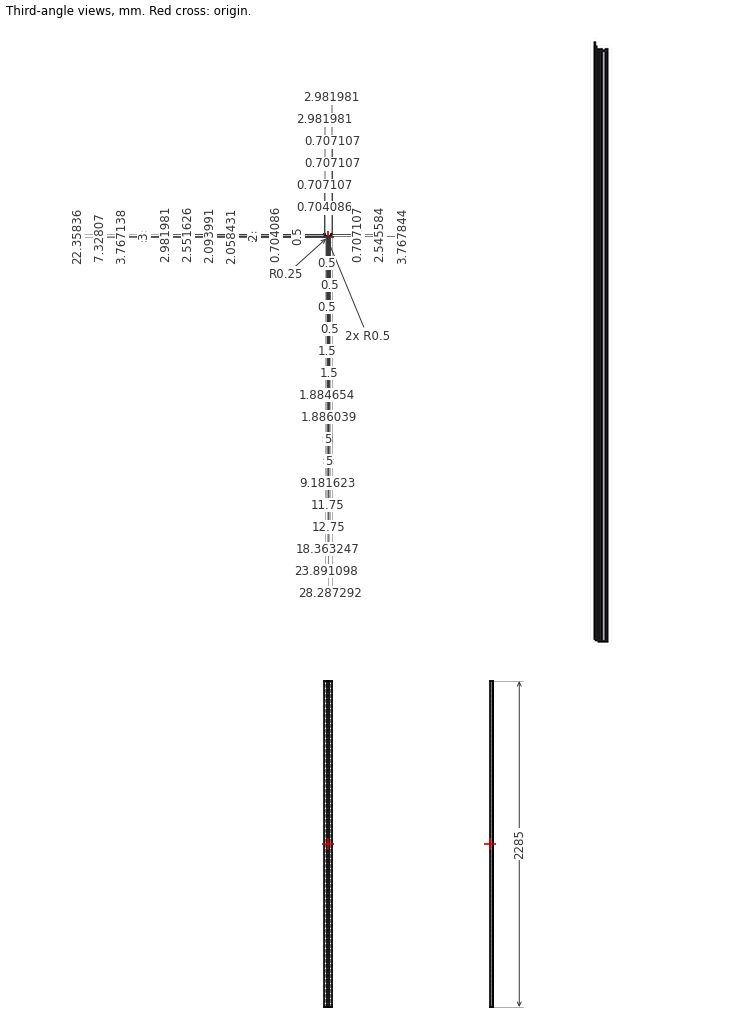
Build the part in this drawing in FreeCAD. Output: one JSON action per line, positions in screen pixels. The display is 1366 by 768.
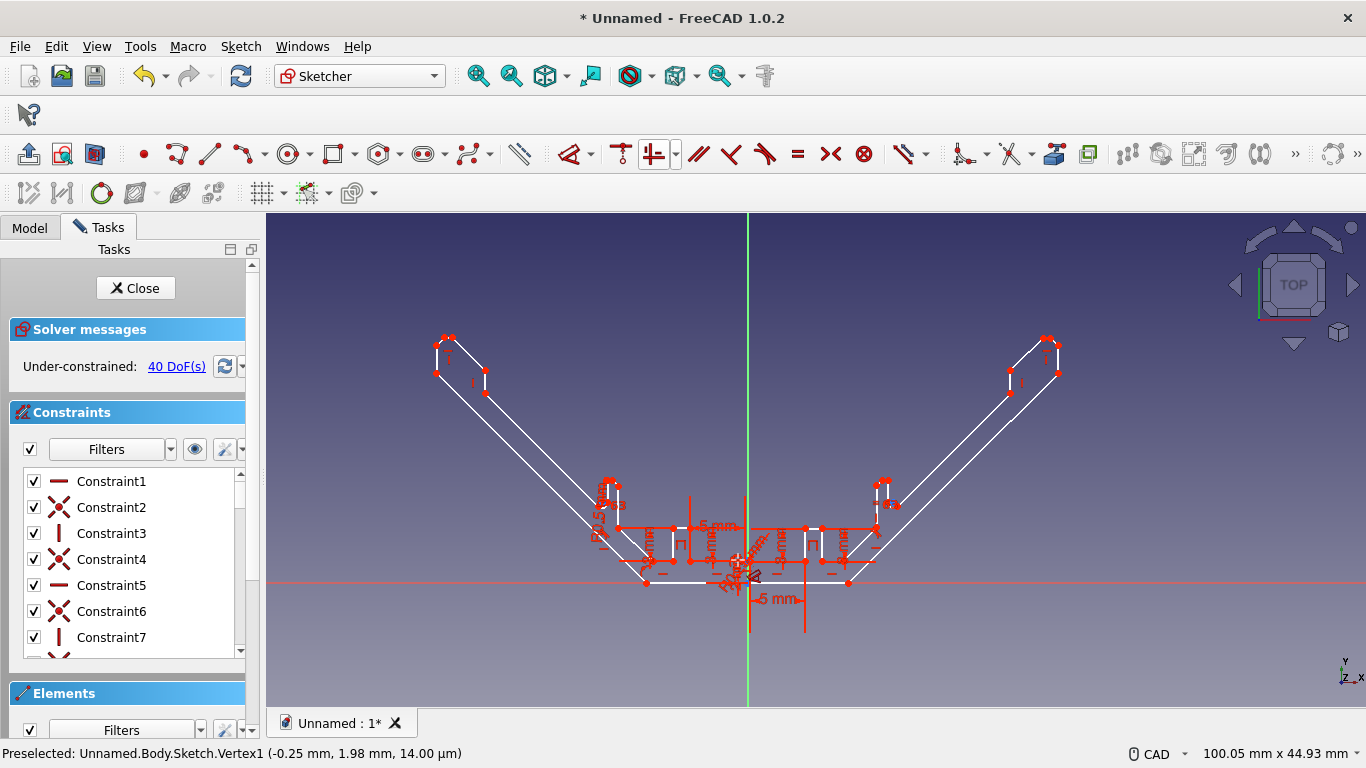
{"action": "scroll", "coordinate": [843, 562], "scroll_direction": "up", "scroll_amount": 3}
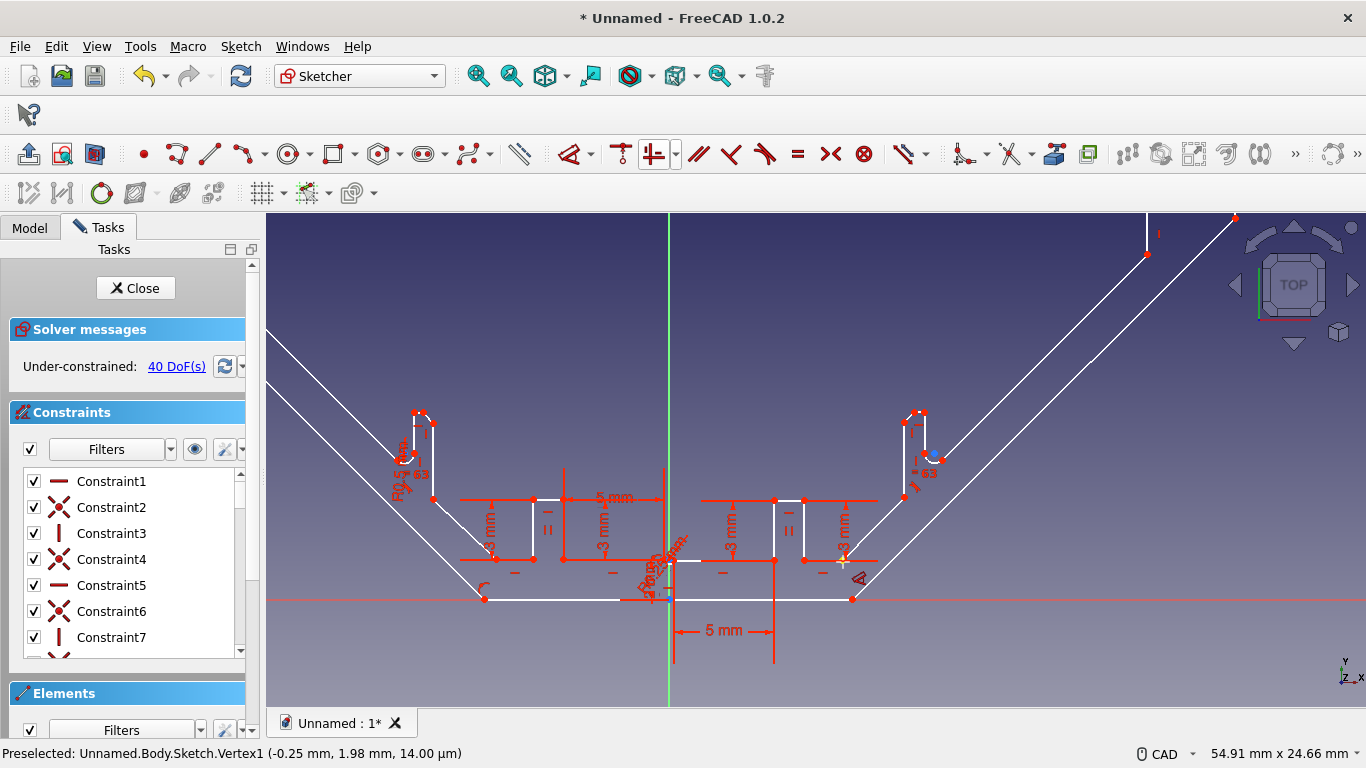
{"action": "left_click", "coordinate": [843, 561]}
{"action": "left_click", "coordinate": [901, 580]}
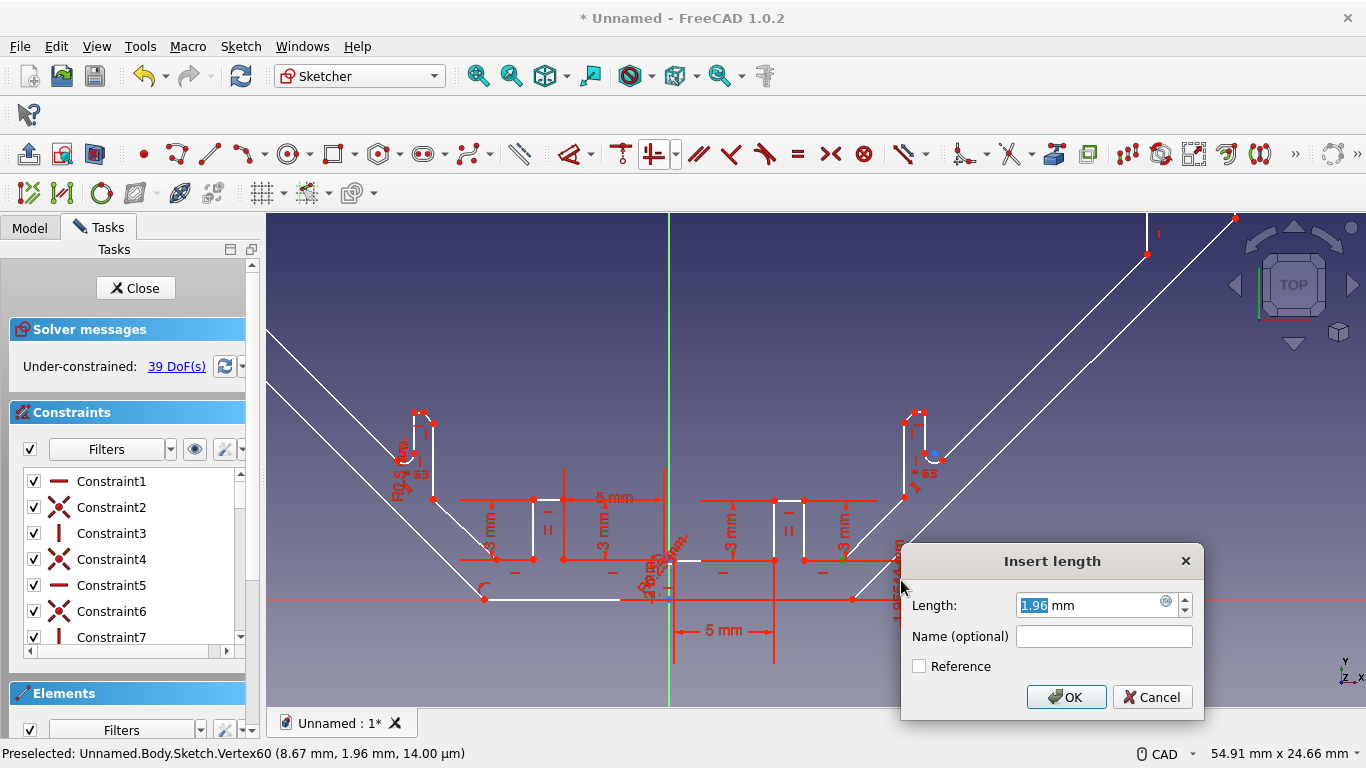
{"action": "type", "text": "2"}
{"action": "key", "text": "Return"}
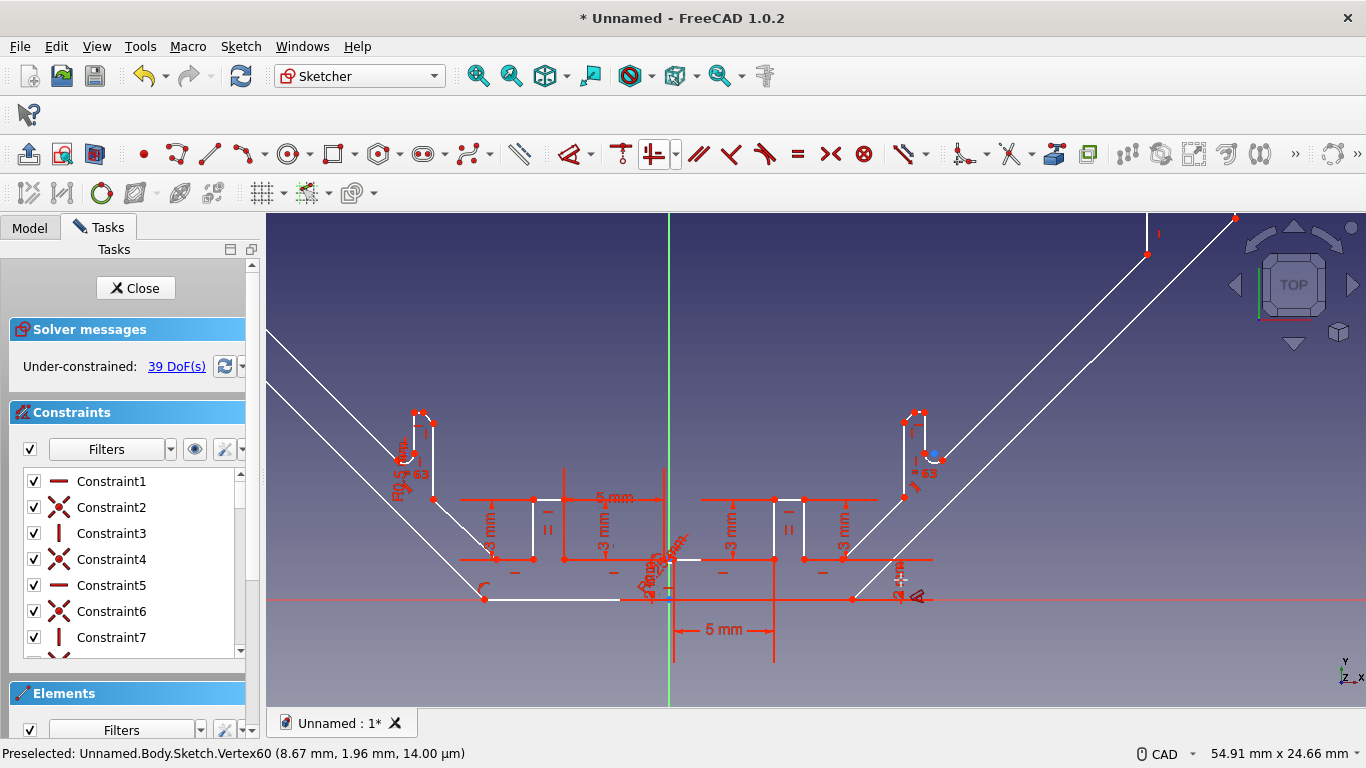
{"action": "scroll", "coordinate": [669, 558], "scroll_direction": "up", "scroll_amount": 5}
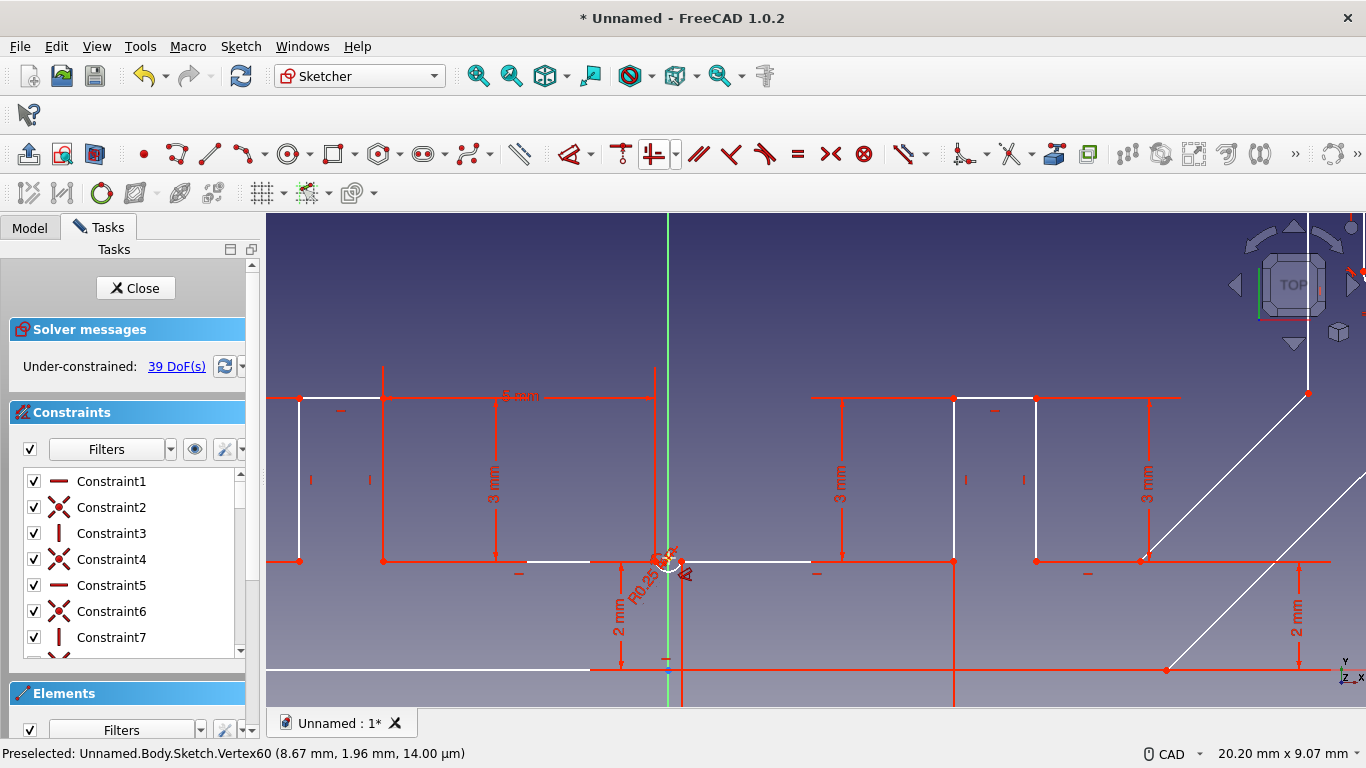
{"action": "left_click", "coordinate": [668, 558]}
{"action": "left_click", "coordinate": [634, 640]}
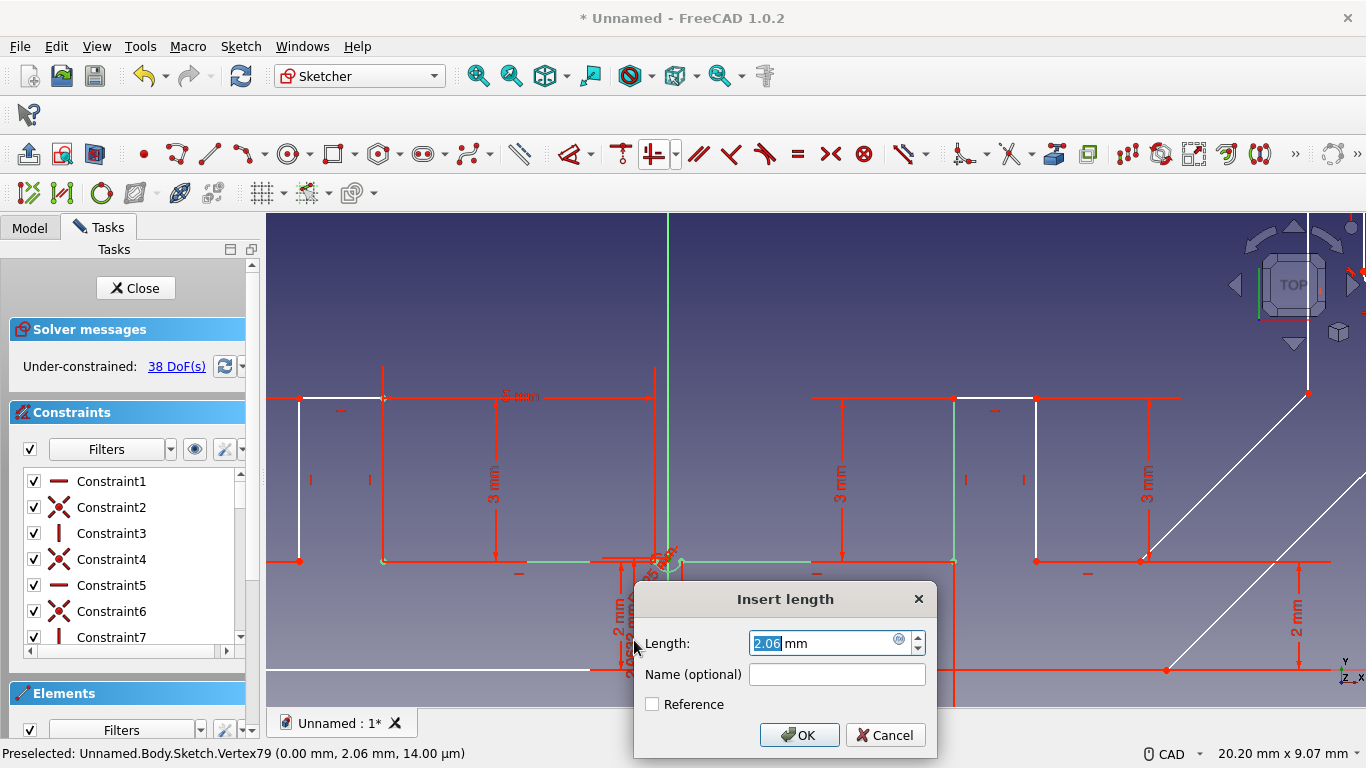
{"action": "type", "text": "2"}
{"action": "key", "text": "Return"}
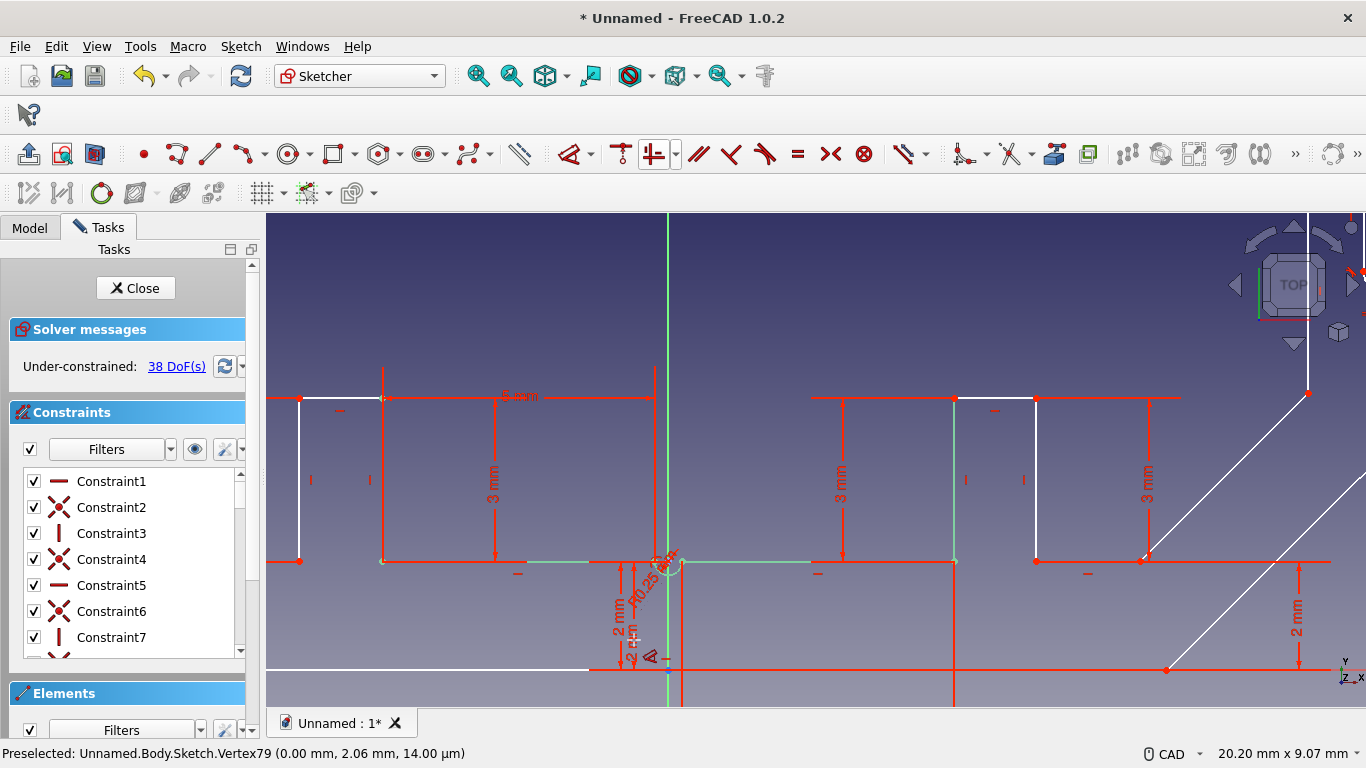
{"action": "left_click", "coordinate": [358, 398]}
{"action": "left_click", "coordinate": [341, 432]}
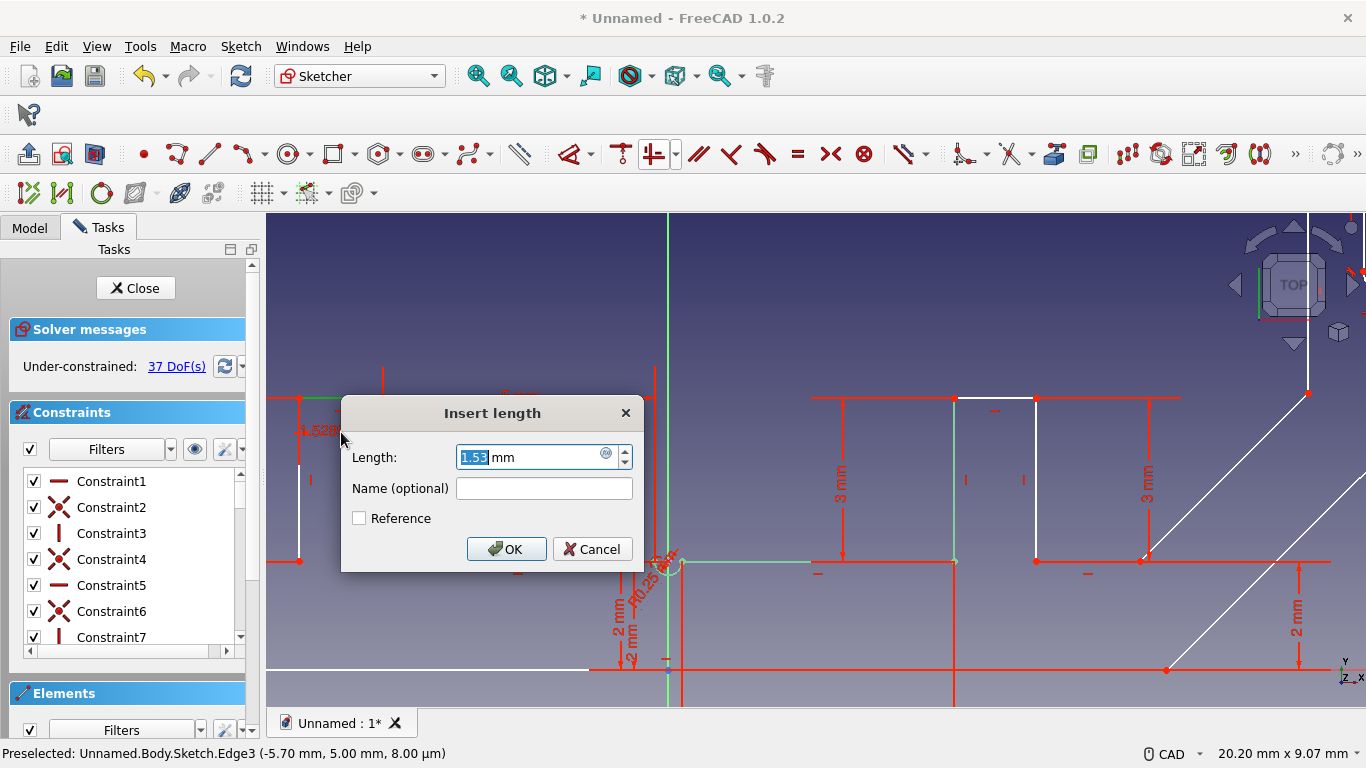
{"action": "type", "text": "1.5"}
{"action": "key", "text": "Return"}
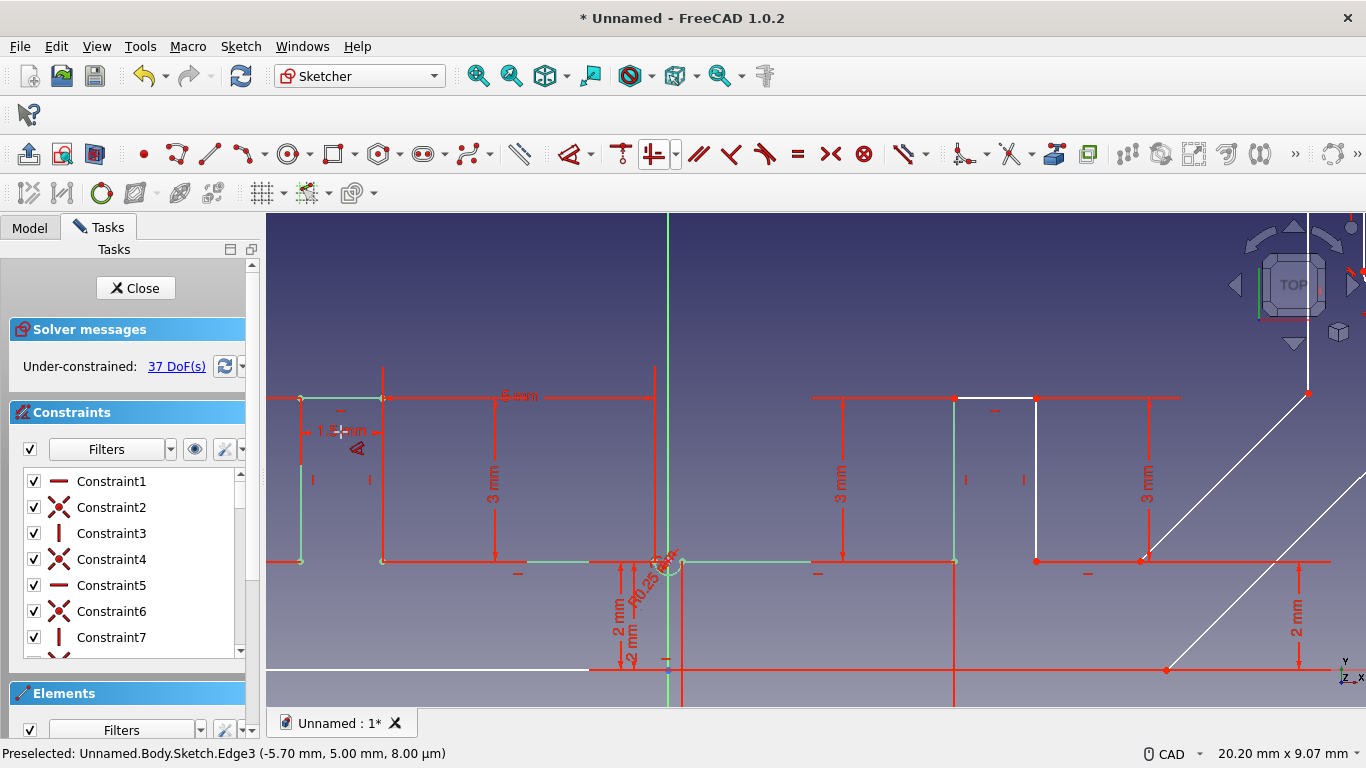
{"action": "scroll", "coordinate": [767, 561], "scroll_direction": "down", "scroll_amount": 8}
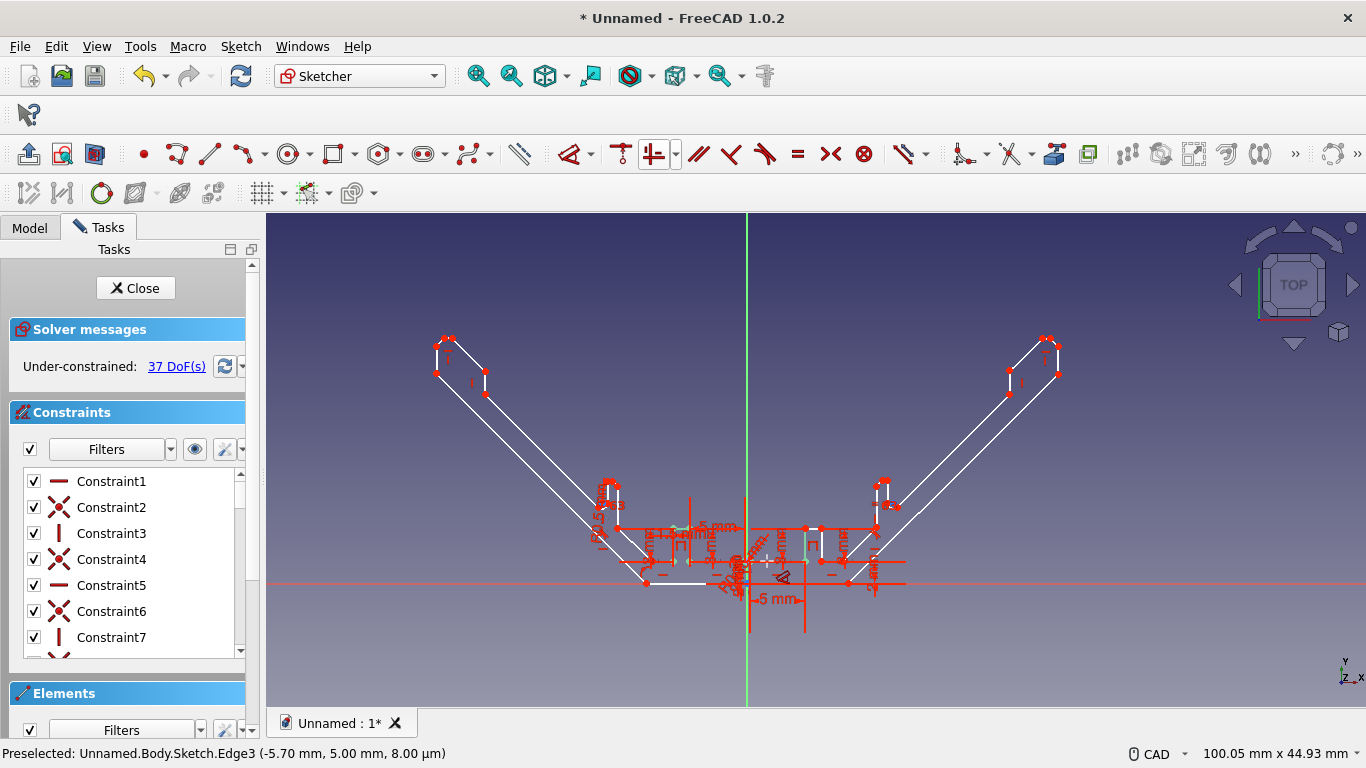
{"action": "scroll", "coordinate": [611, 481], "scroll_direction": "up", "scroll_amount": 10}